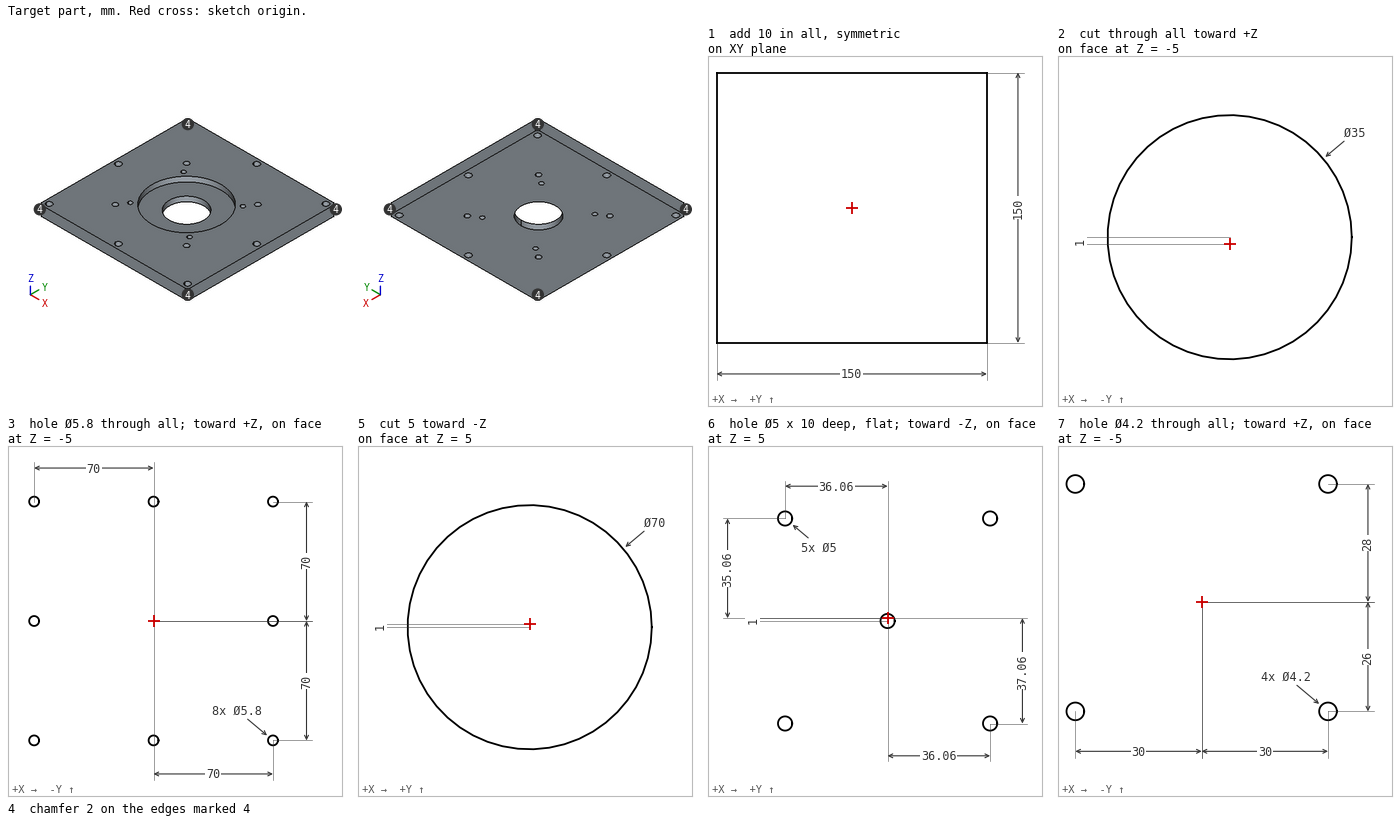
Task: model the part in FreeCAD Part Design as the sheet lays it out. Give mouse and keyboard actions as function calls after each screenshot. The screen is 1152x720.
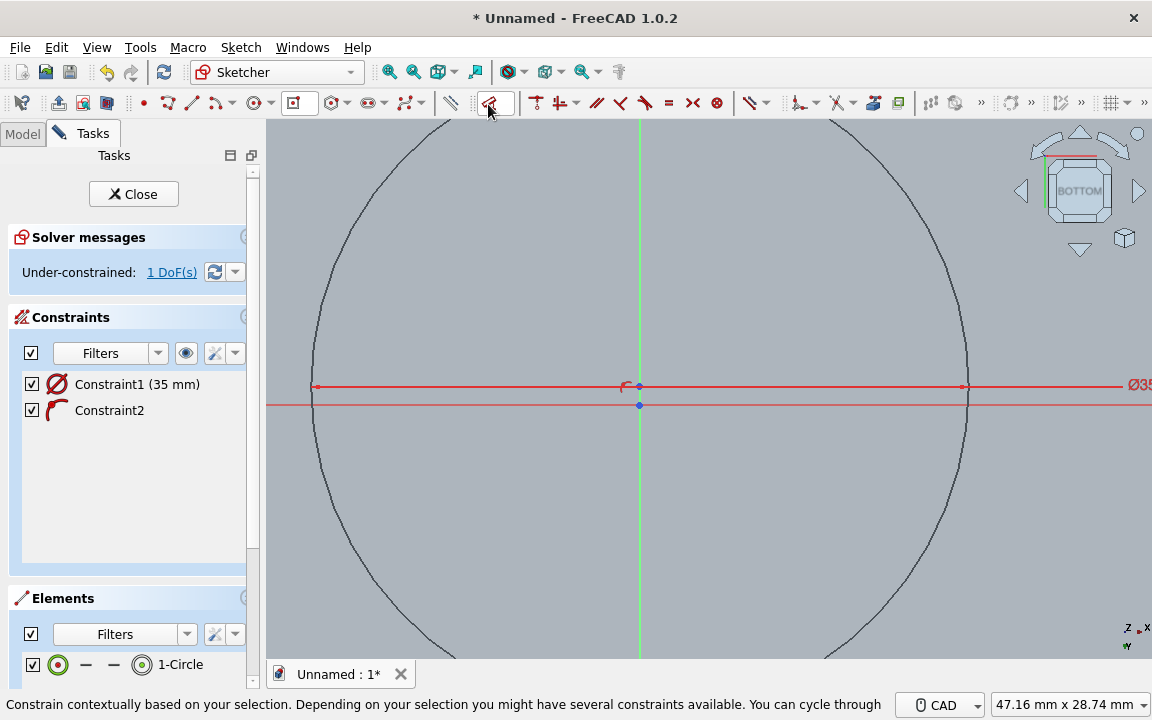
scroll(640, 387, up, 4)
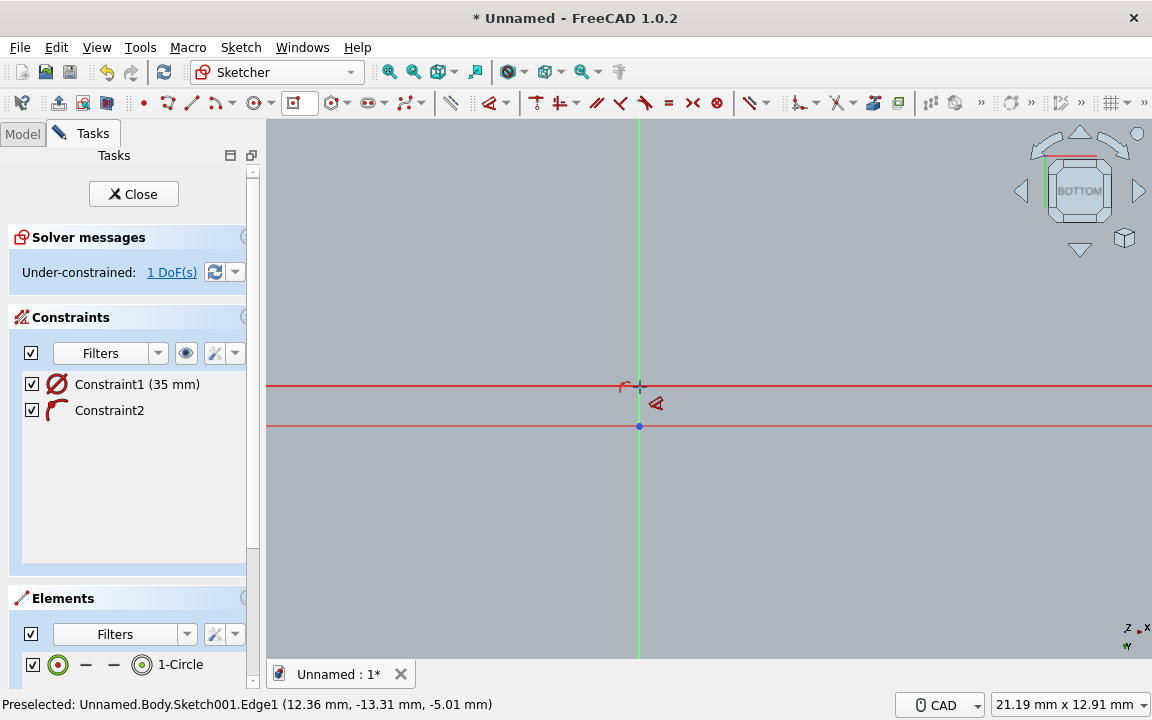
click(639, 386)
click(673, 406)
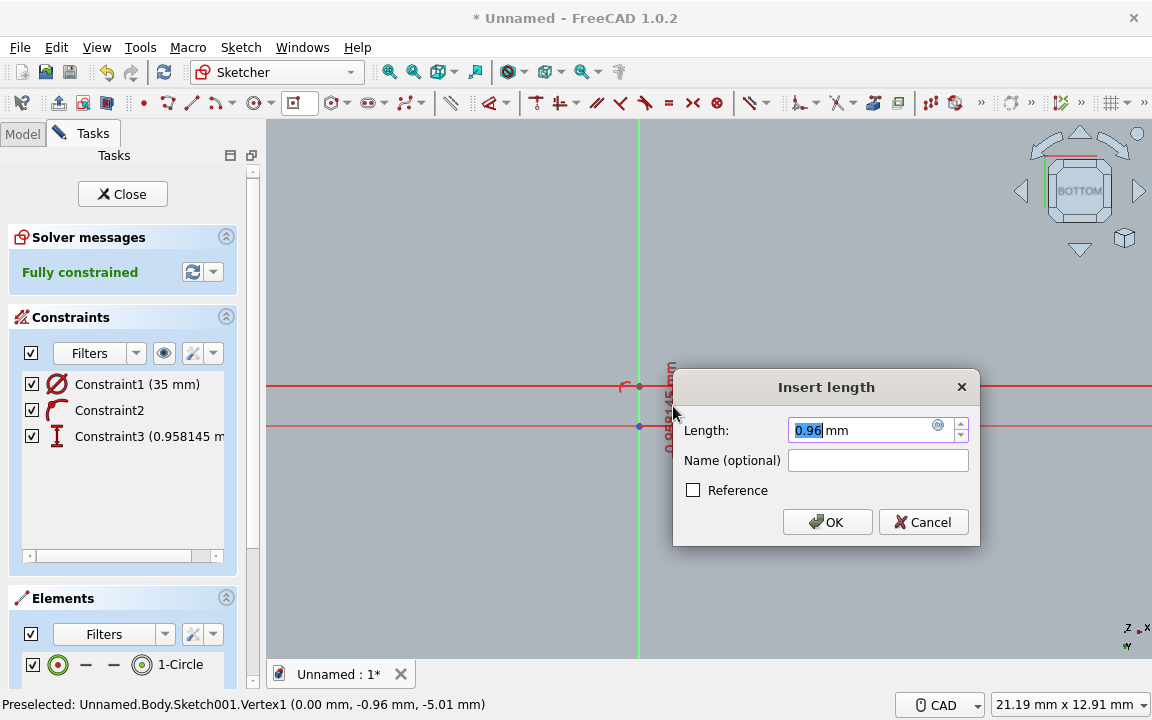
text(1)
key(Return)
key(Escape)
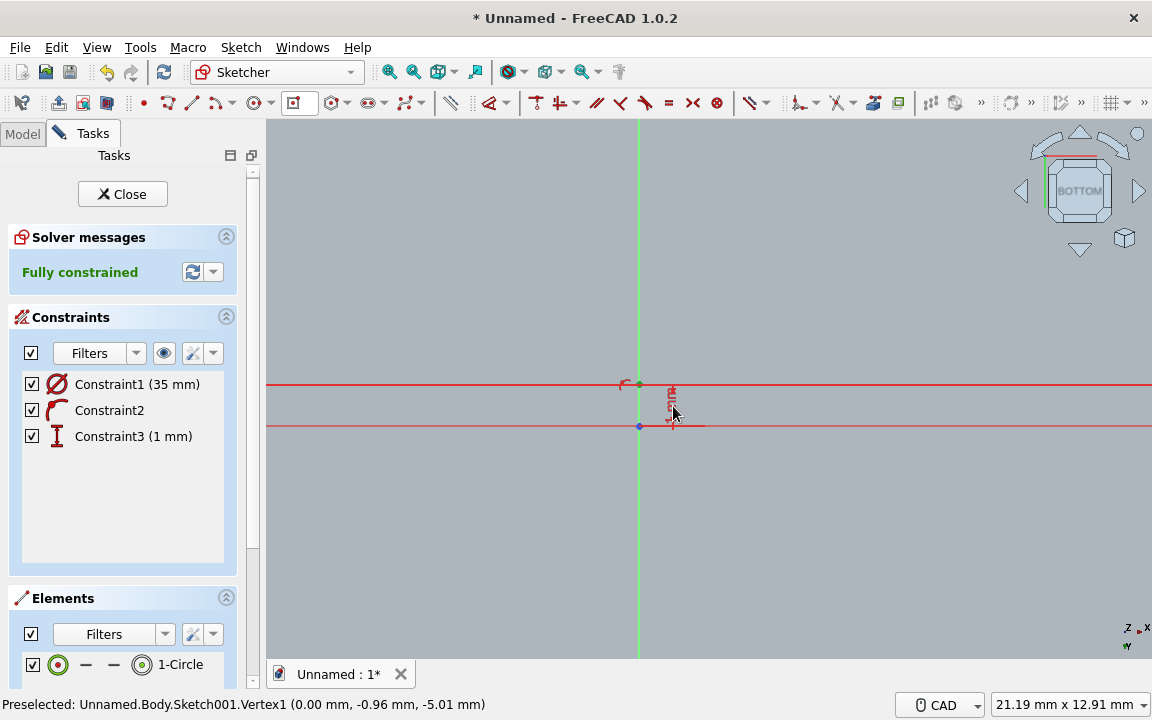
click(123, 194)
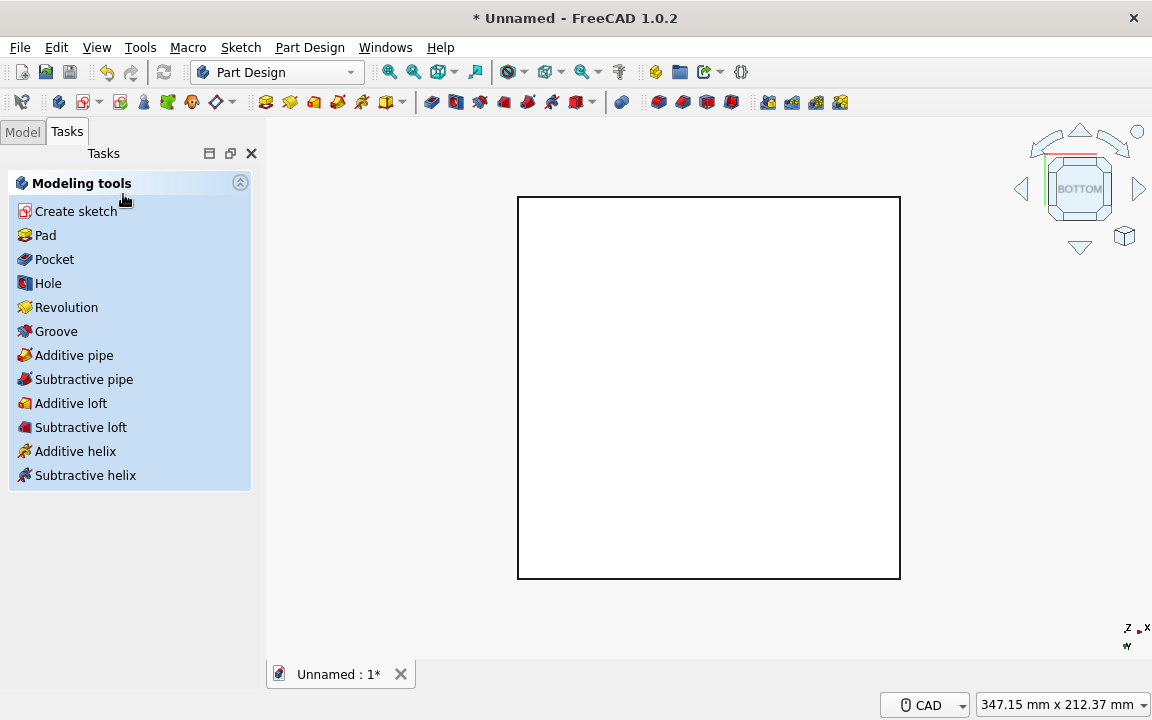
click(432, 102)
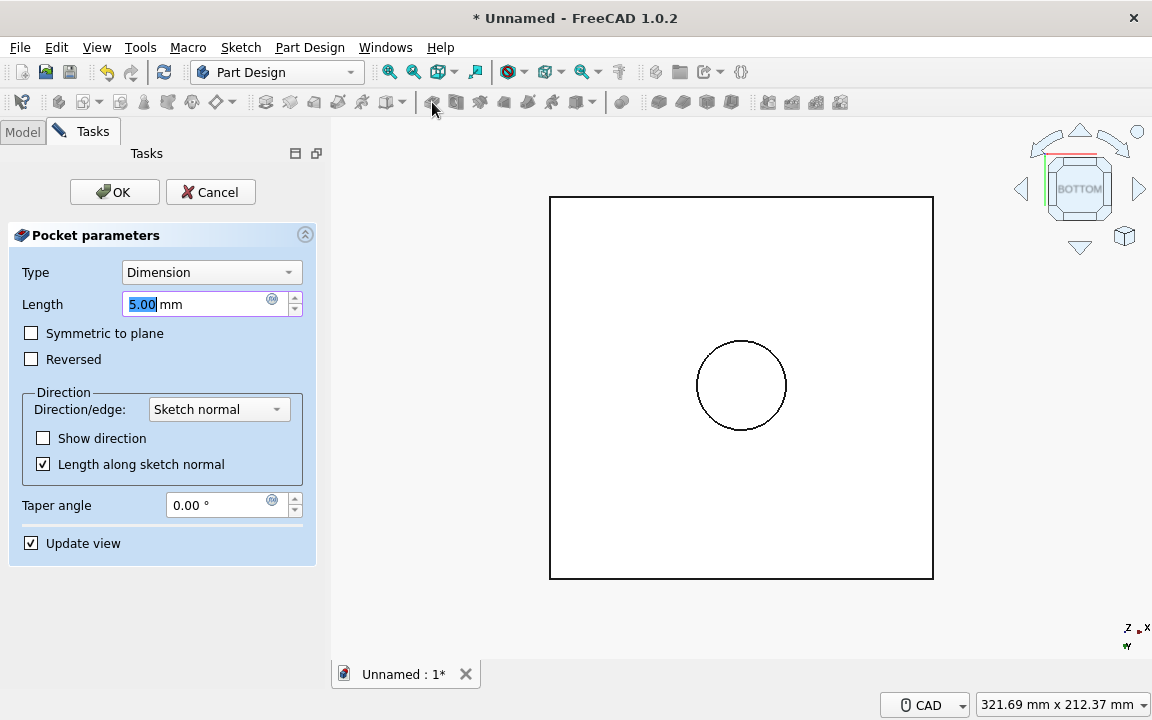
click(212, 272)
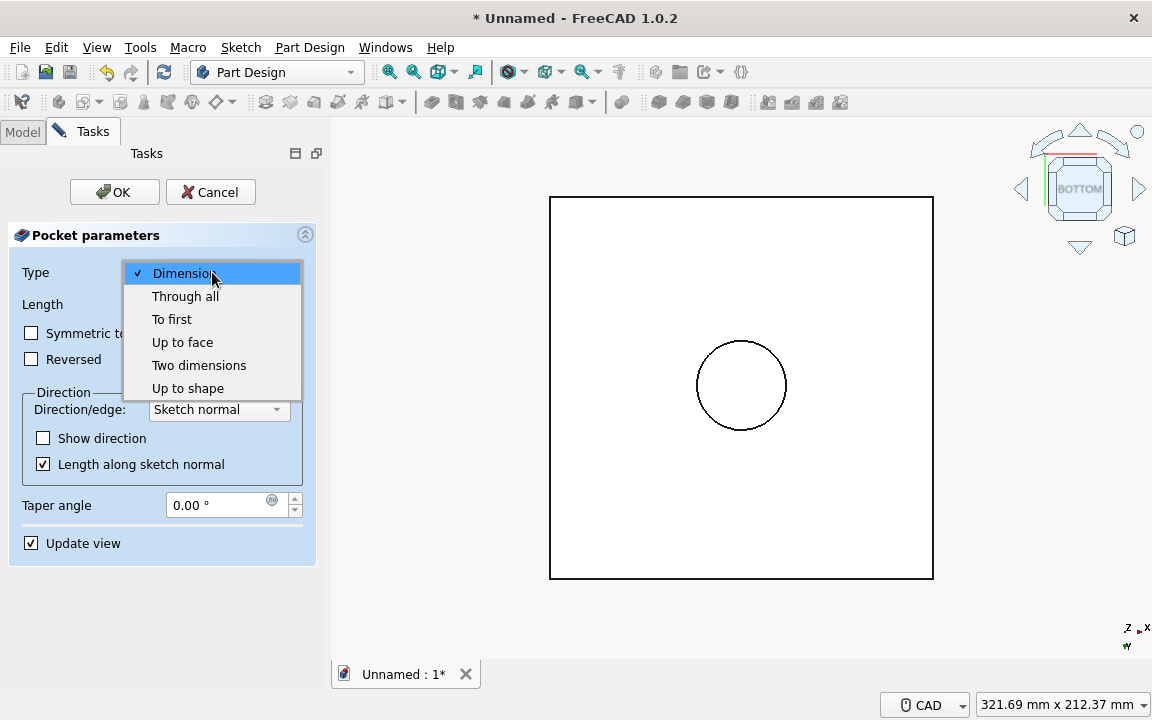
click(212, 296)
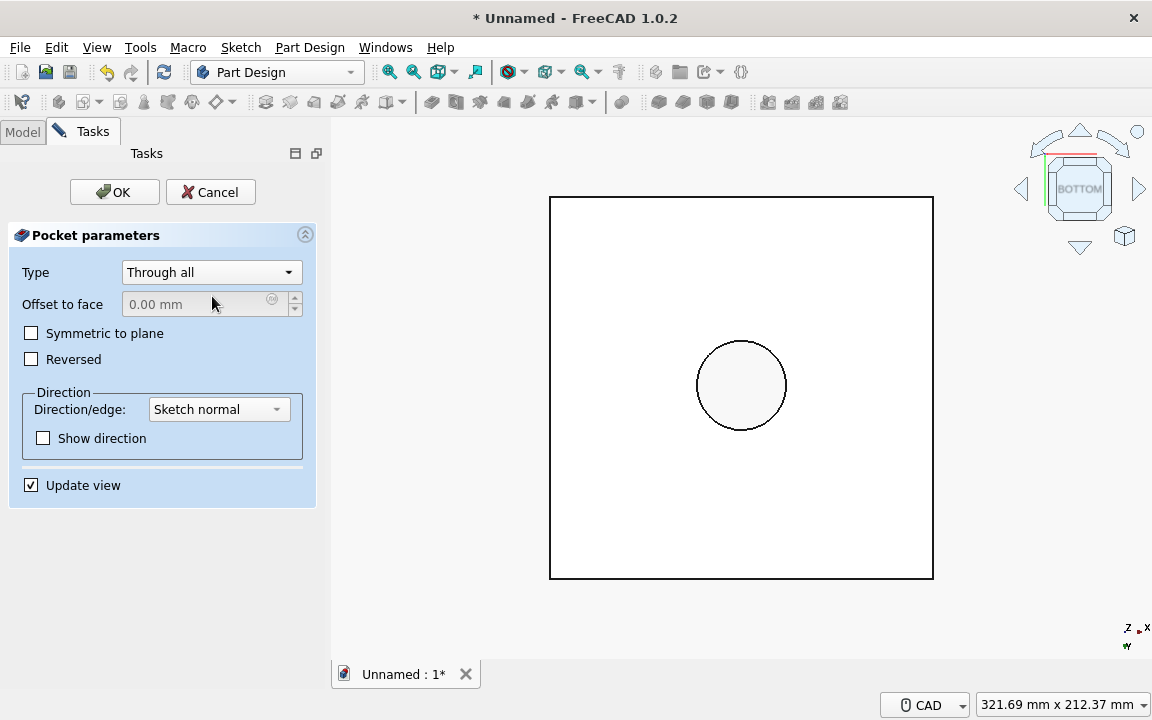
click(115, 192)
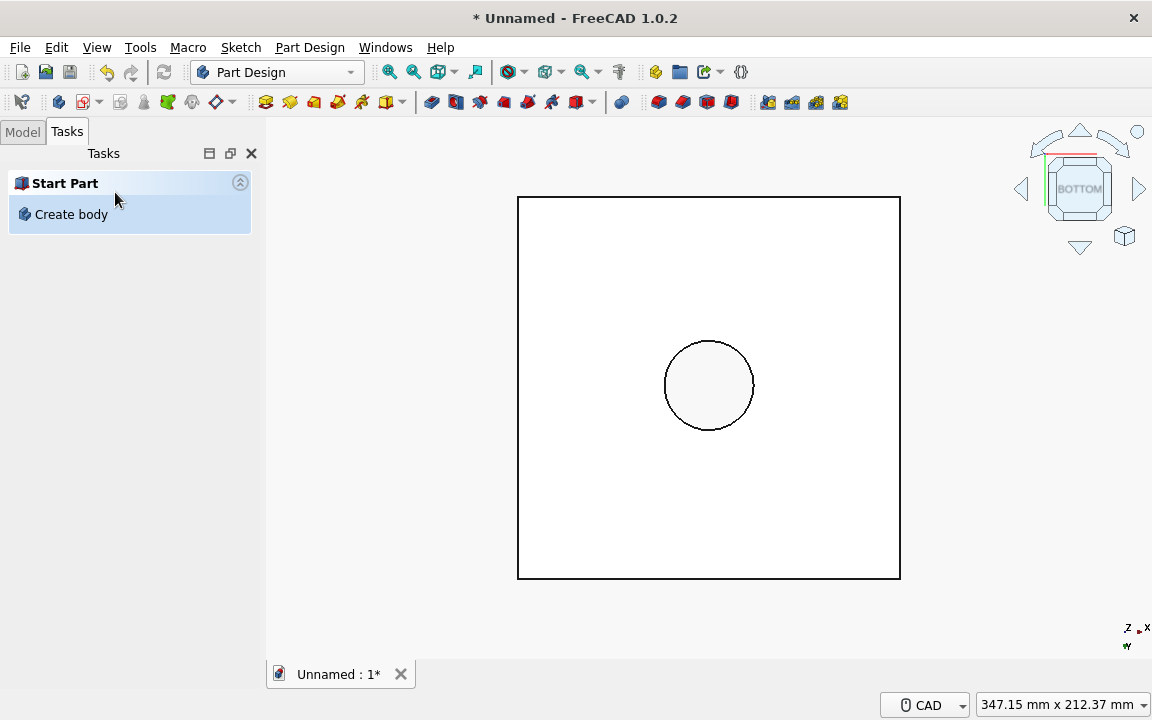
click(600, 278)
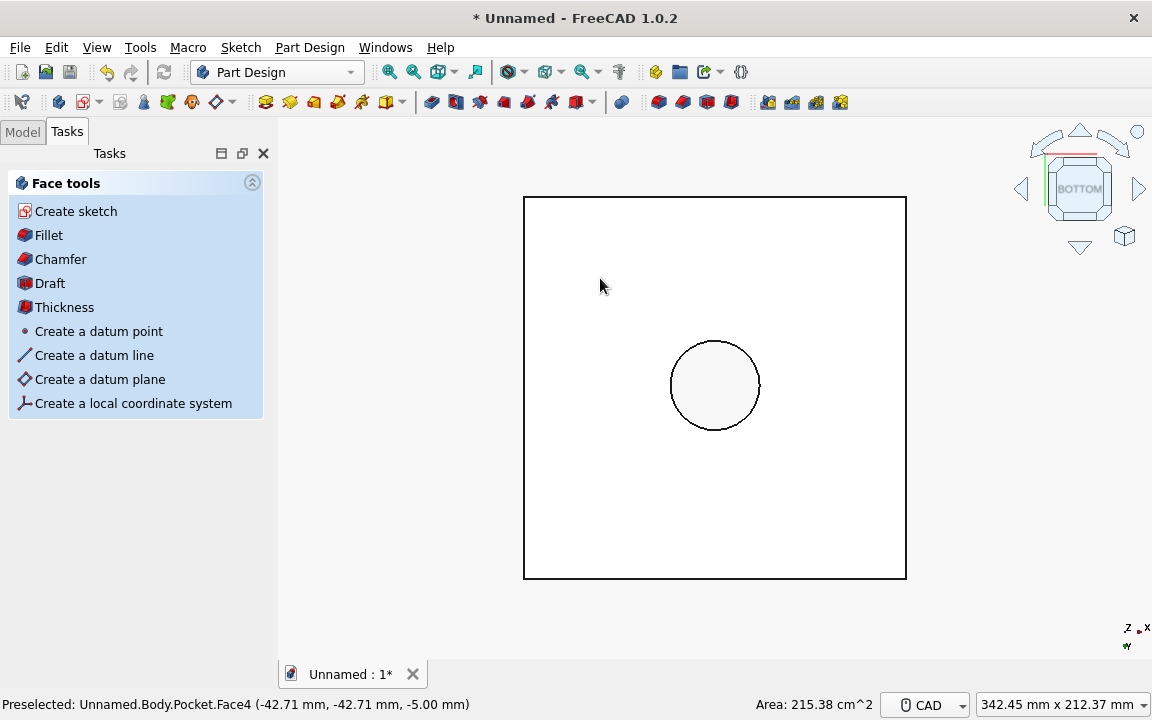
click(84, 102)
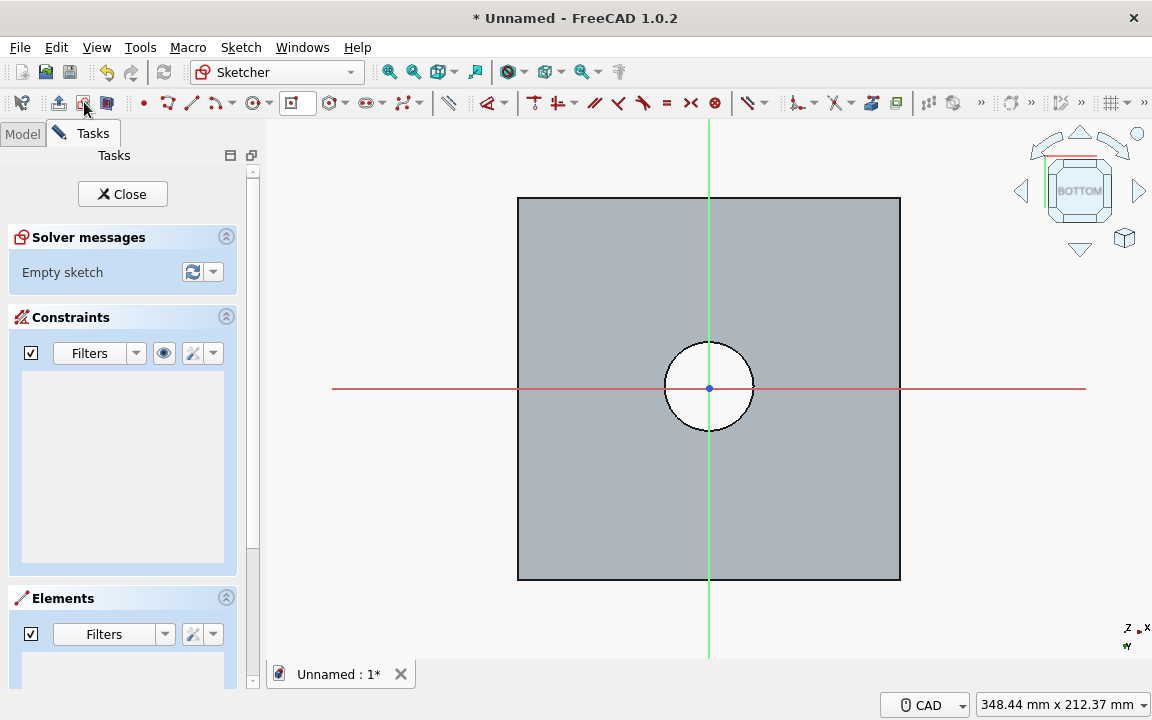
click(254, 104)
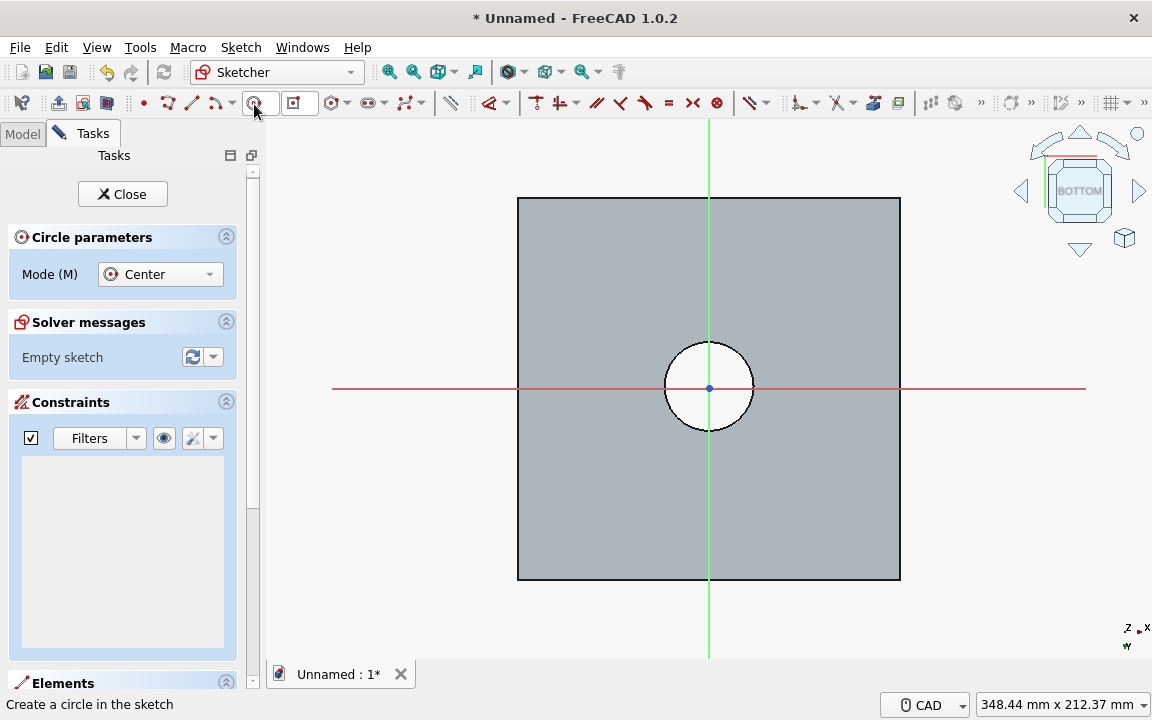
scroll(887, 567, up, 6)